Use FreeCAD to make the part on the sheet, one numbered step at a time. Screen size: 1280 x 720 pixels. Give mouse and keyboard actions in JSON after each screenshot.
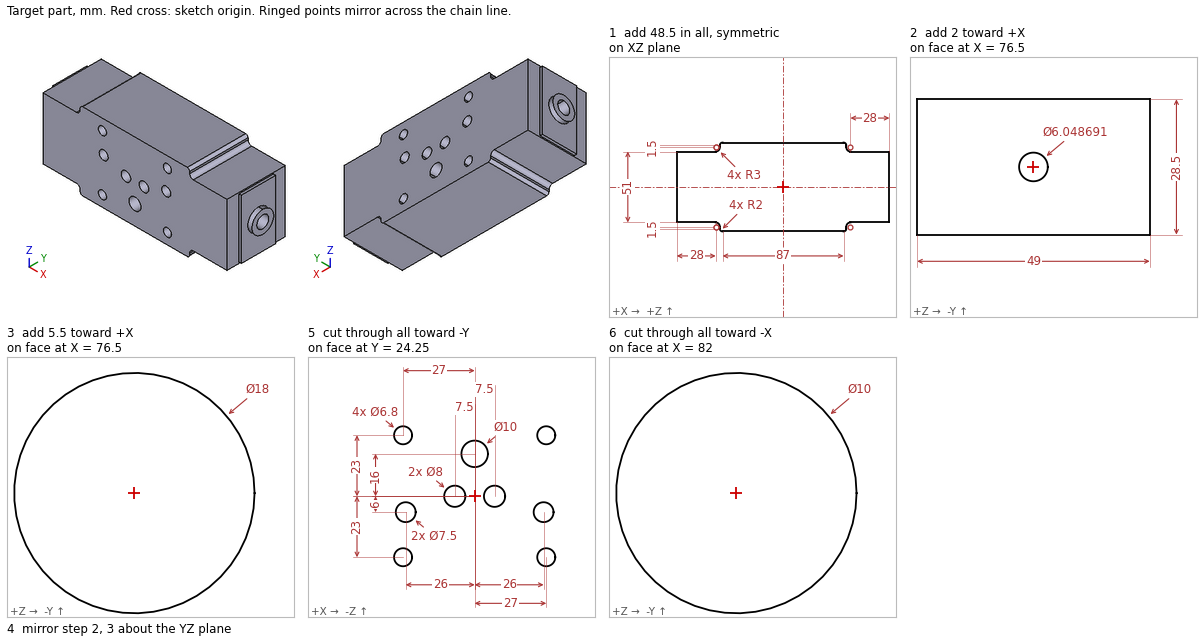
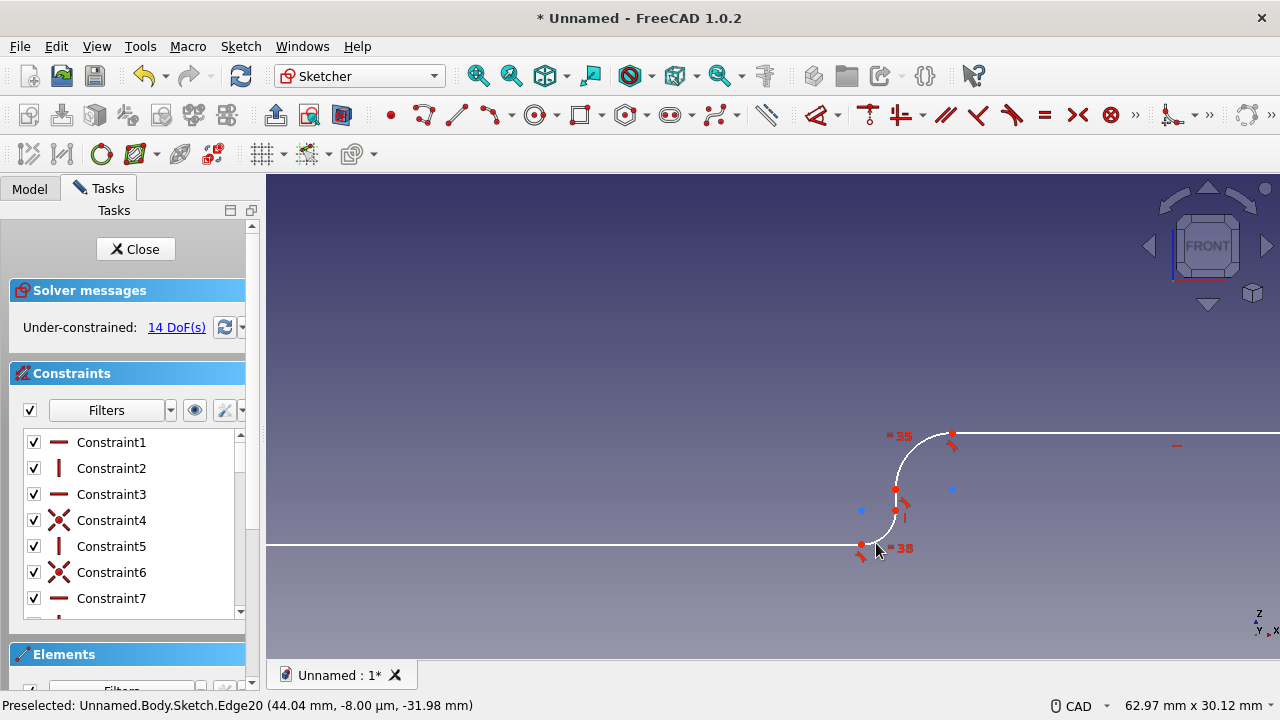
{"action": "scroll", "coordinate": [879, 544], "scroll_direction": "down", "scroll_amount": 7}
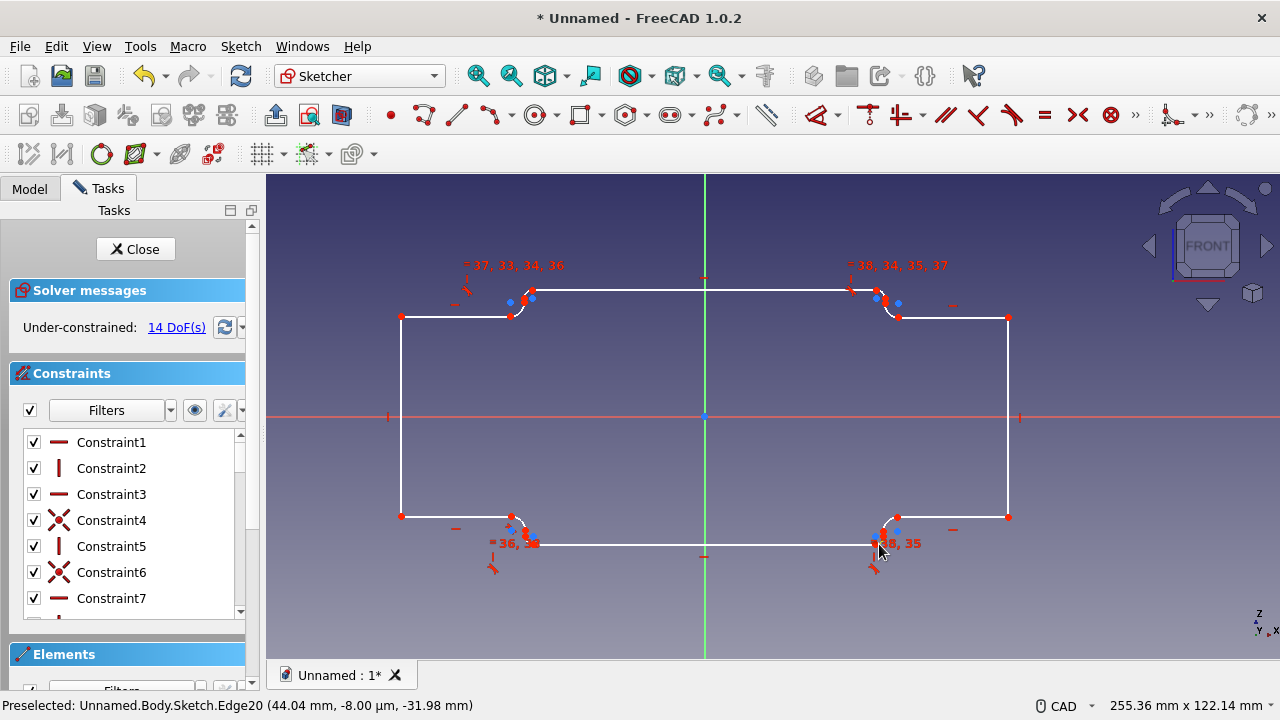
{"action": "left_click", "coordinate": [511, 531]}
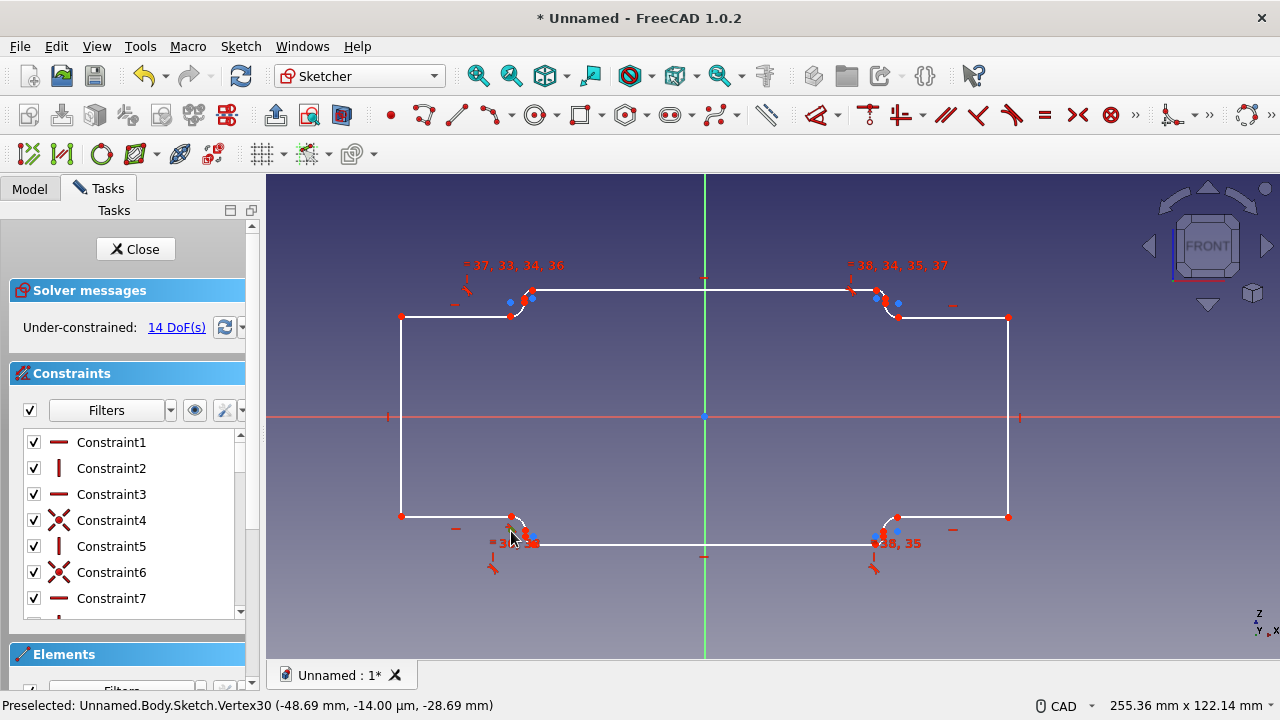
{"action": "left_click", "coordinate": [510, 303]}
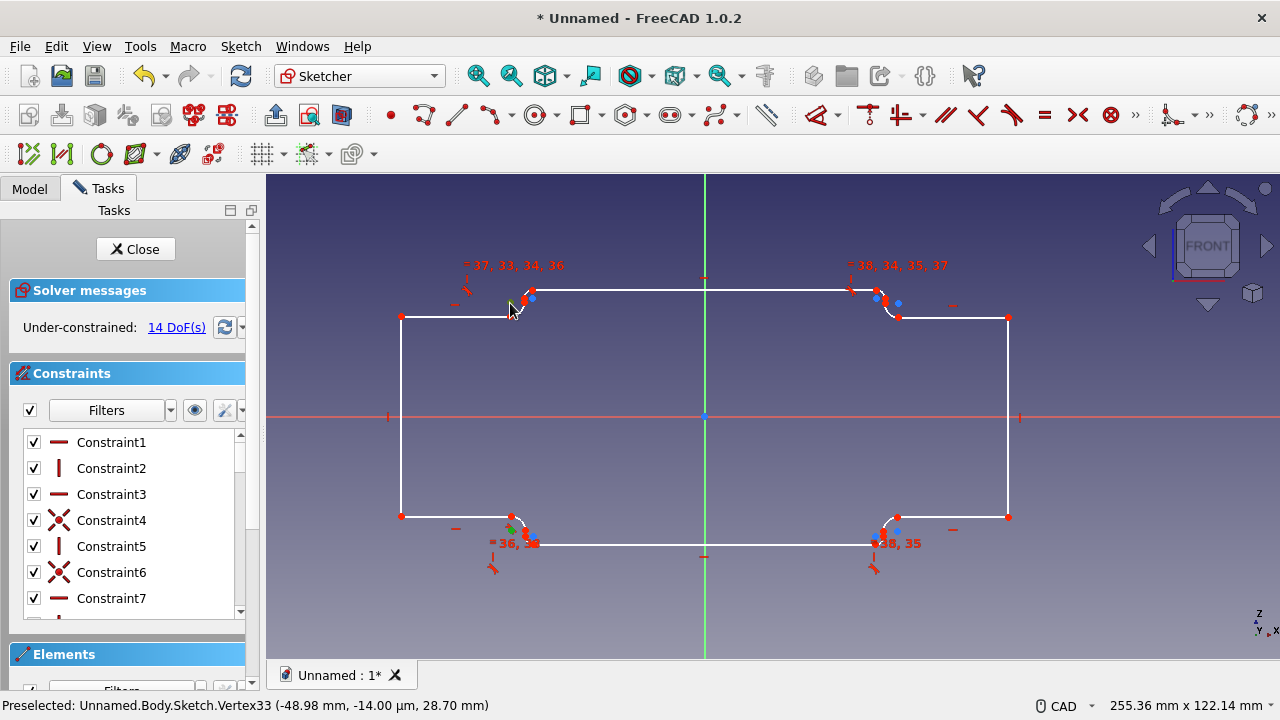
{"action": "left_click", "coordinate": [353, 417]}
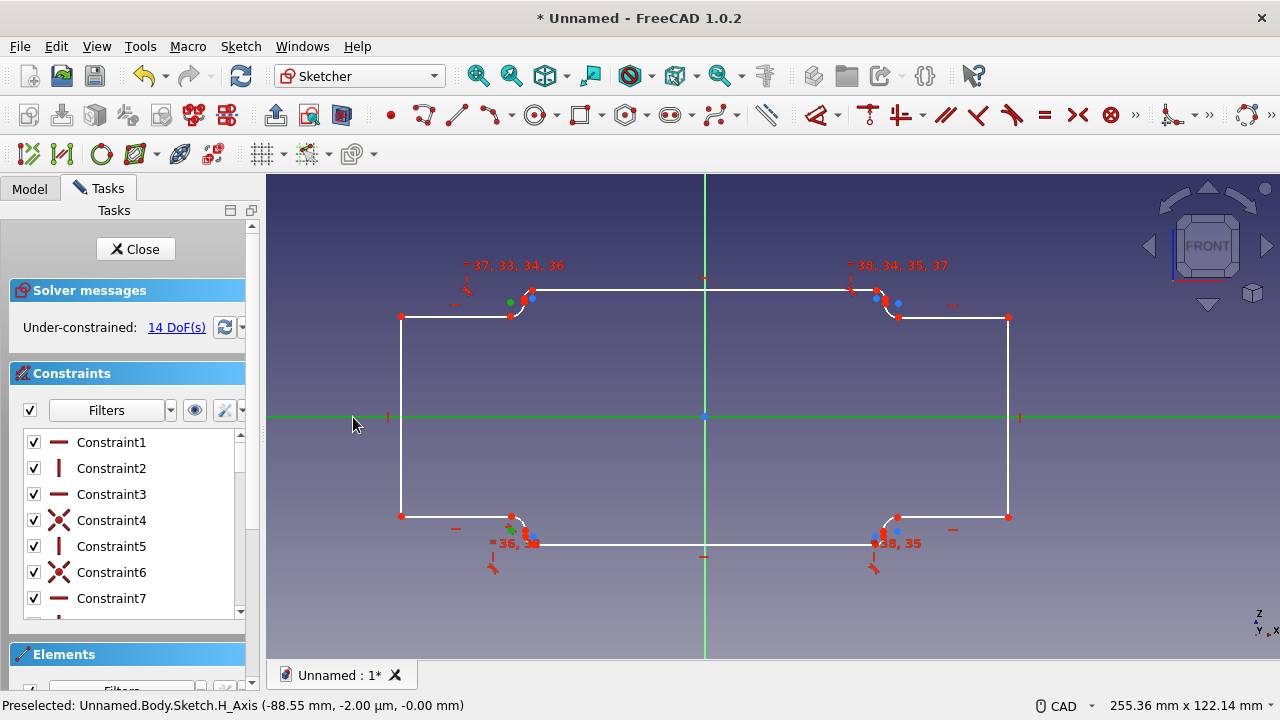
{"action": "left_click", "coordinate": [1078, 116]}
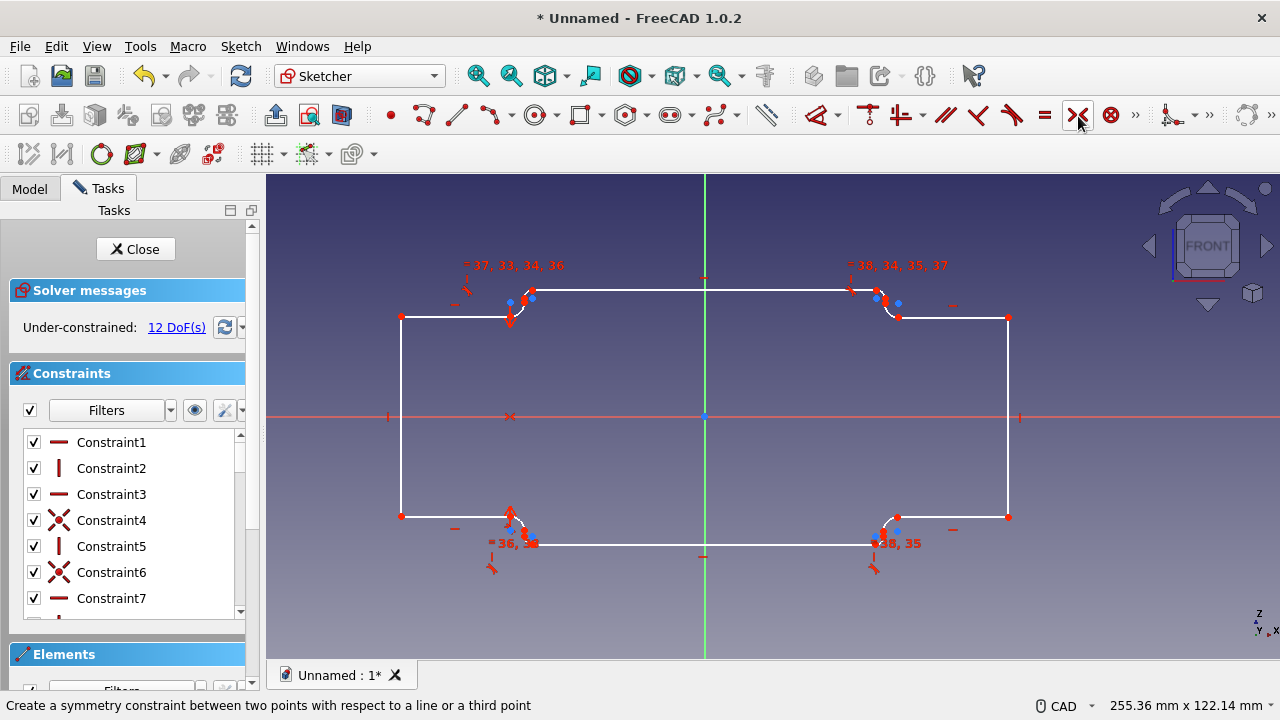
{"action": "left_click", "coordinate": [510, 303]}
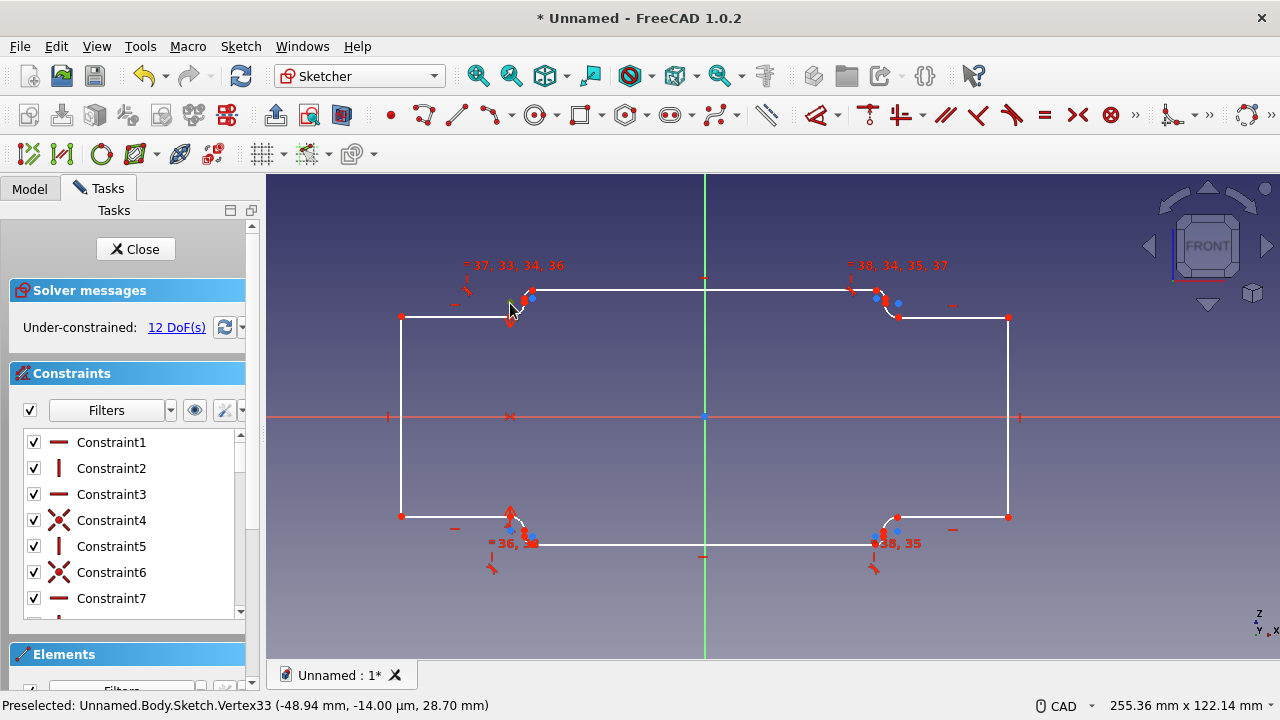
{"action": "left_click", "coordinate": [899, 304]}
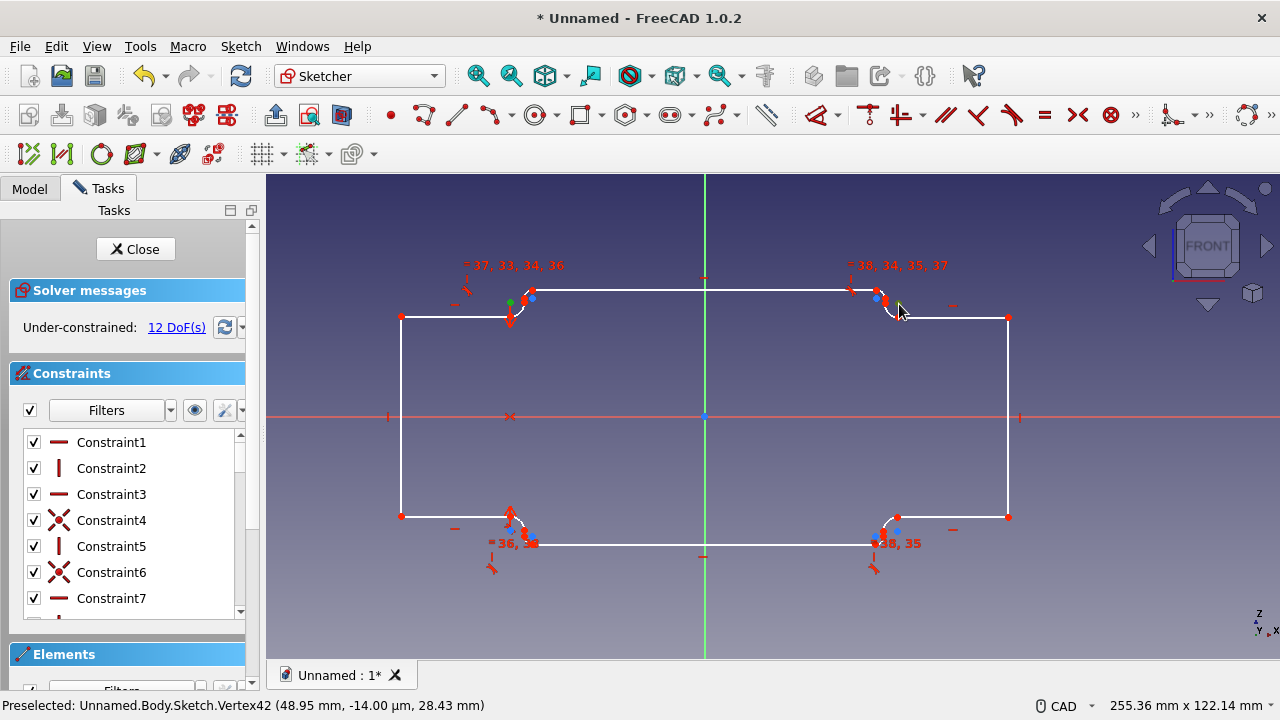
{"action": "left_click", "coordinate": [705, 600]}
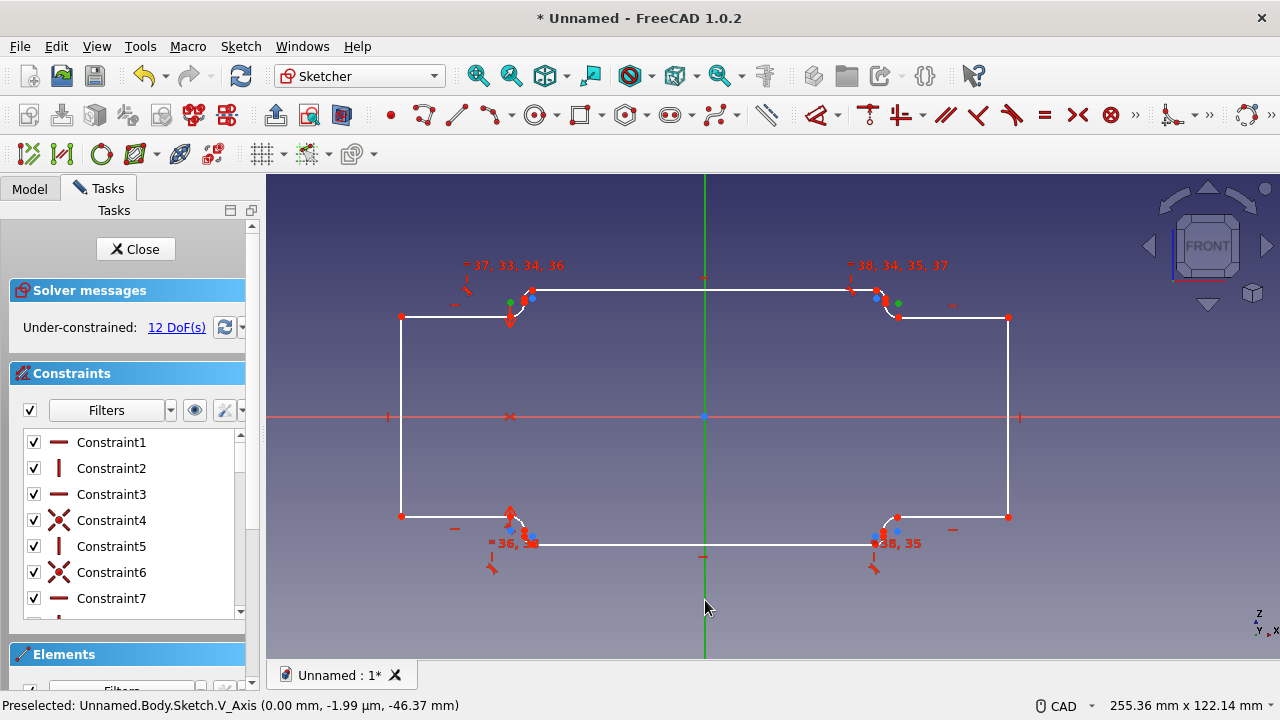
{"action": "left_click", "coordinate": [1078, 116]}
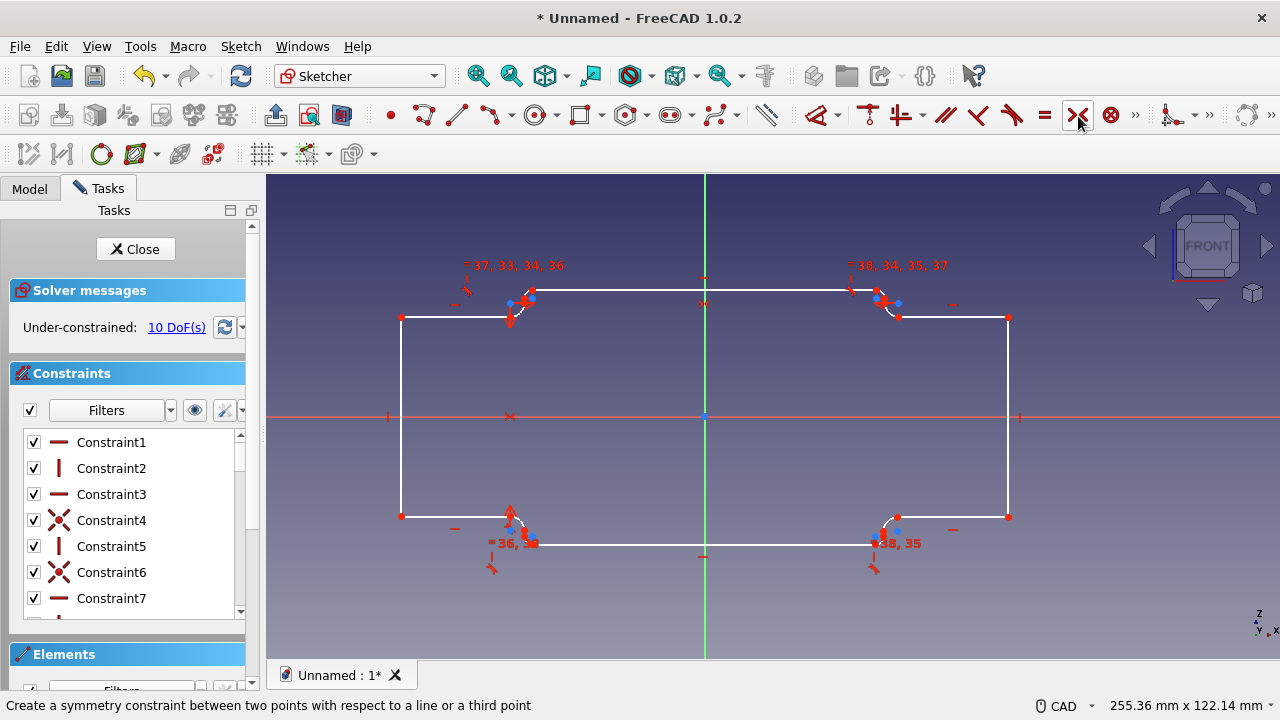
{"action": "left_click", "coordinate": [510, 531]}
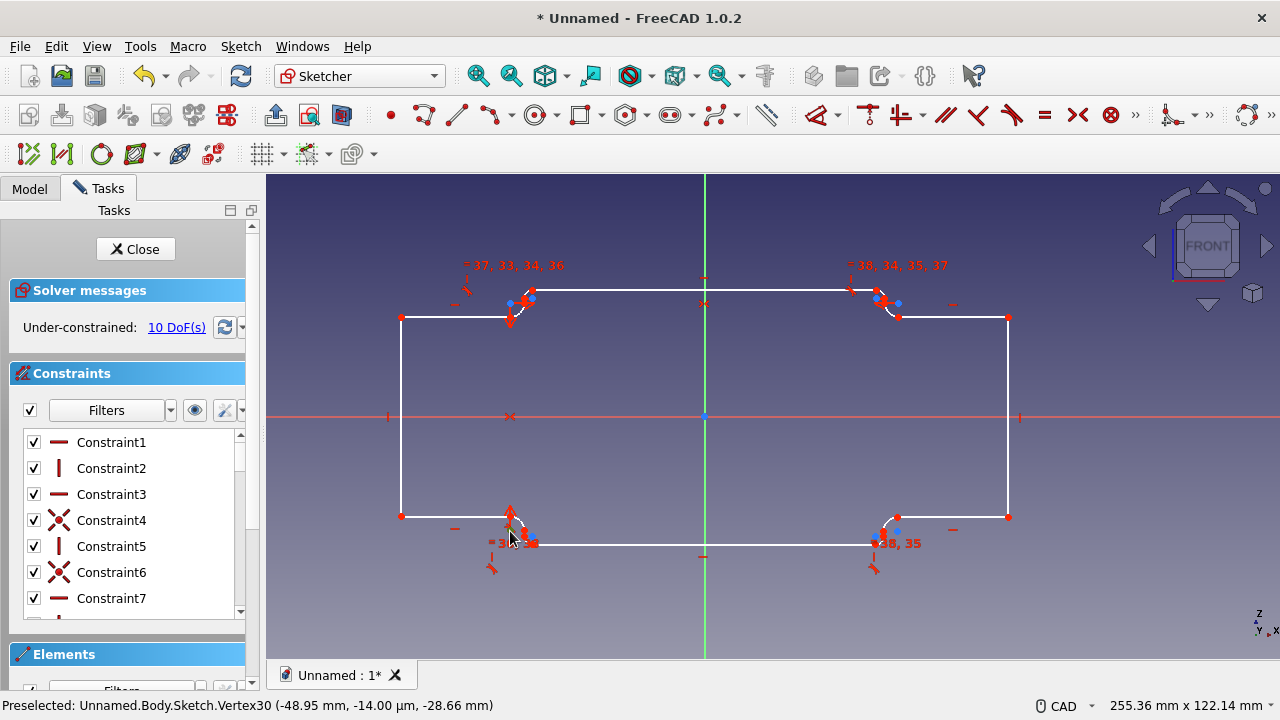
{"action": "left_click", "coordinate": [898, 531]}